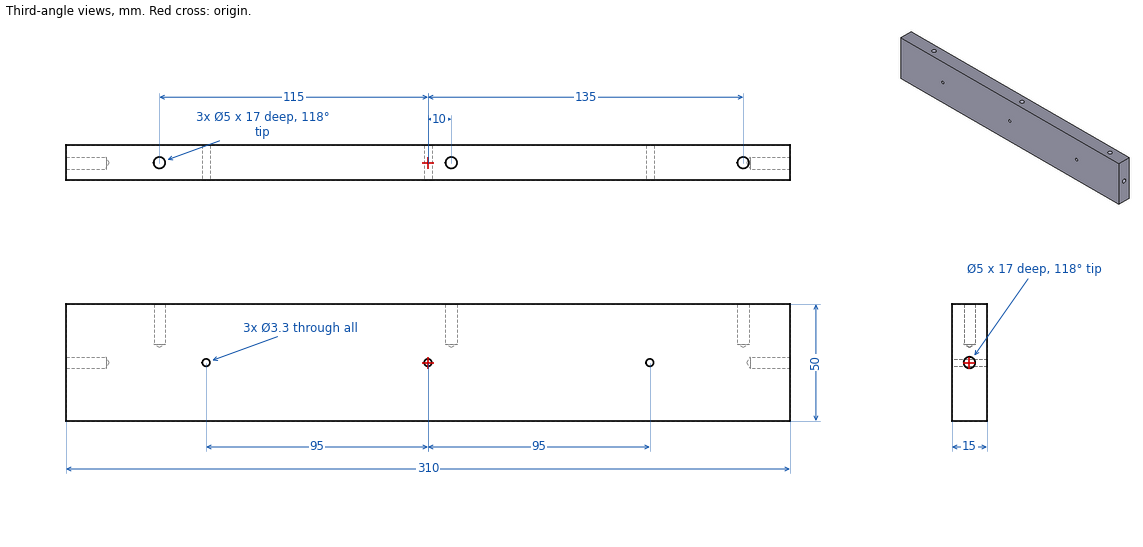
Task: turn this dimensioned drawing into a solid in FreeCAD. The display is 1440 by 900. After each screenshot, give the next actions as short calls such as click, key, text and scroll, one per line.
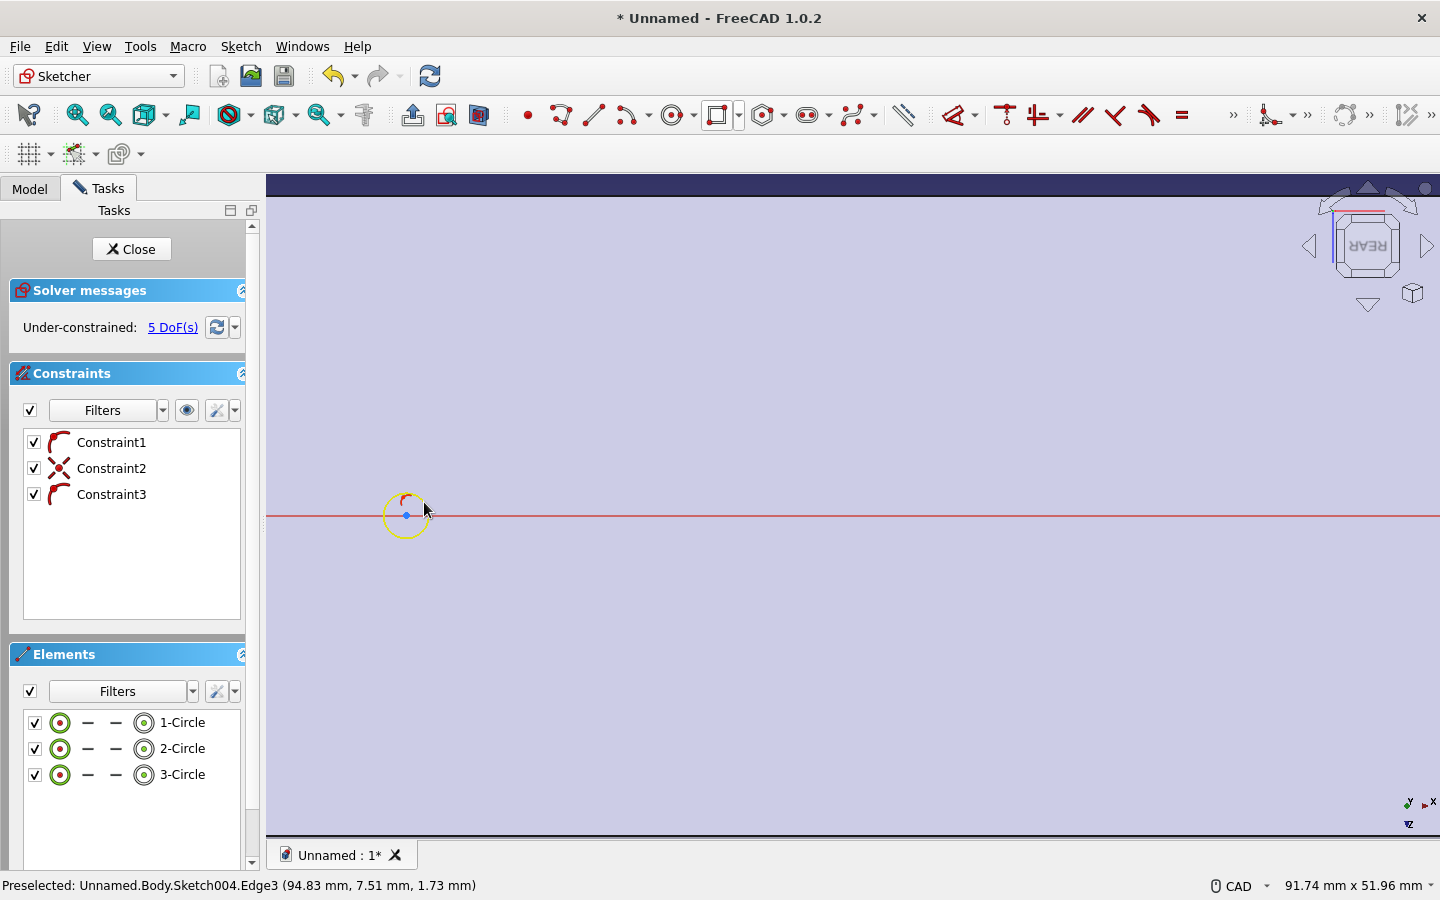
click(422, 500)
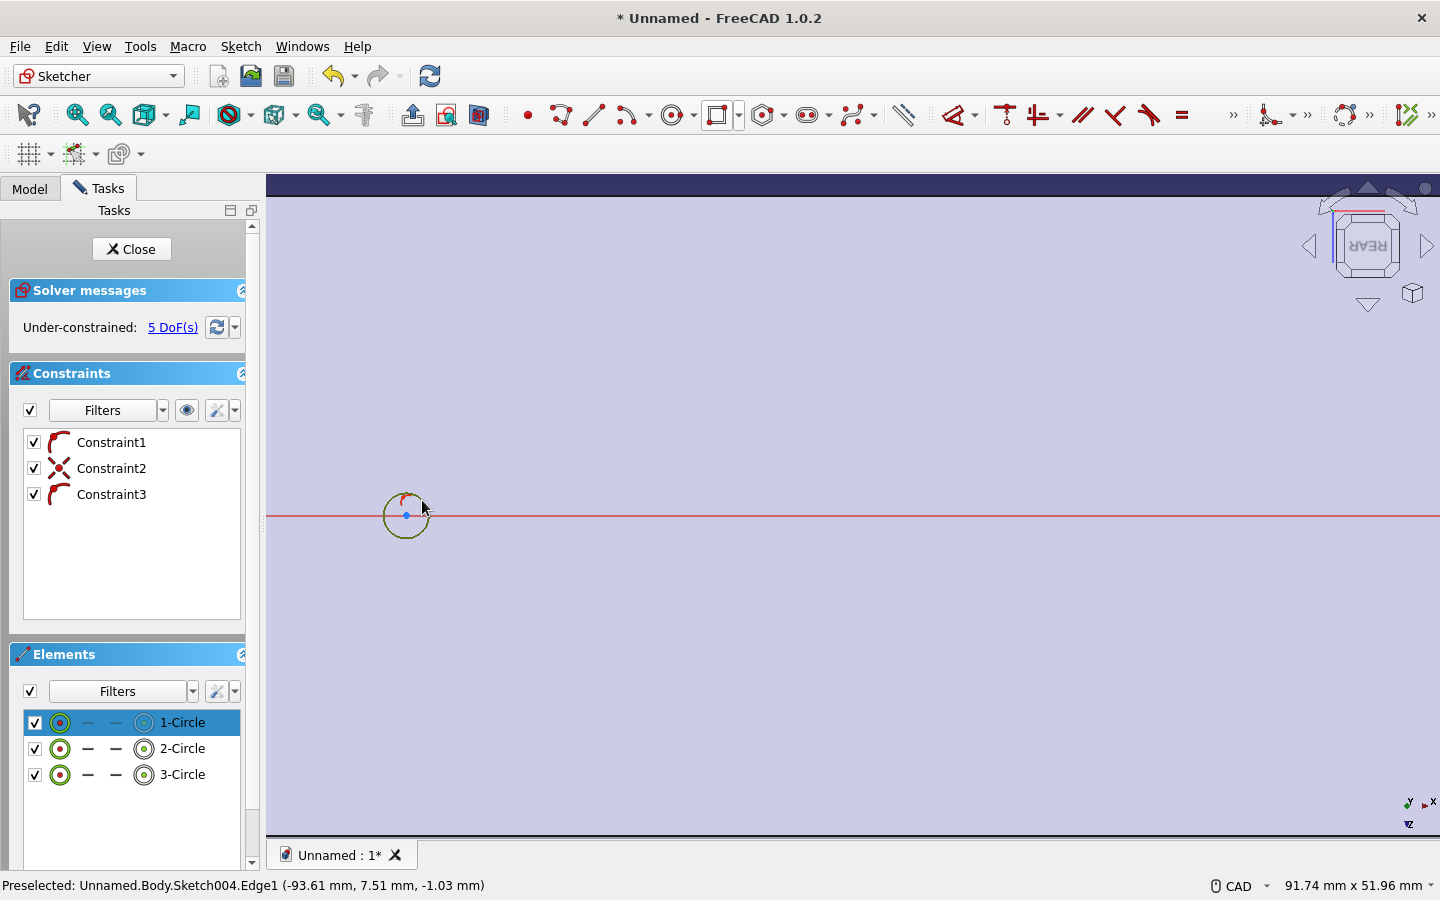
scroll(423, 502, down, 6)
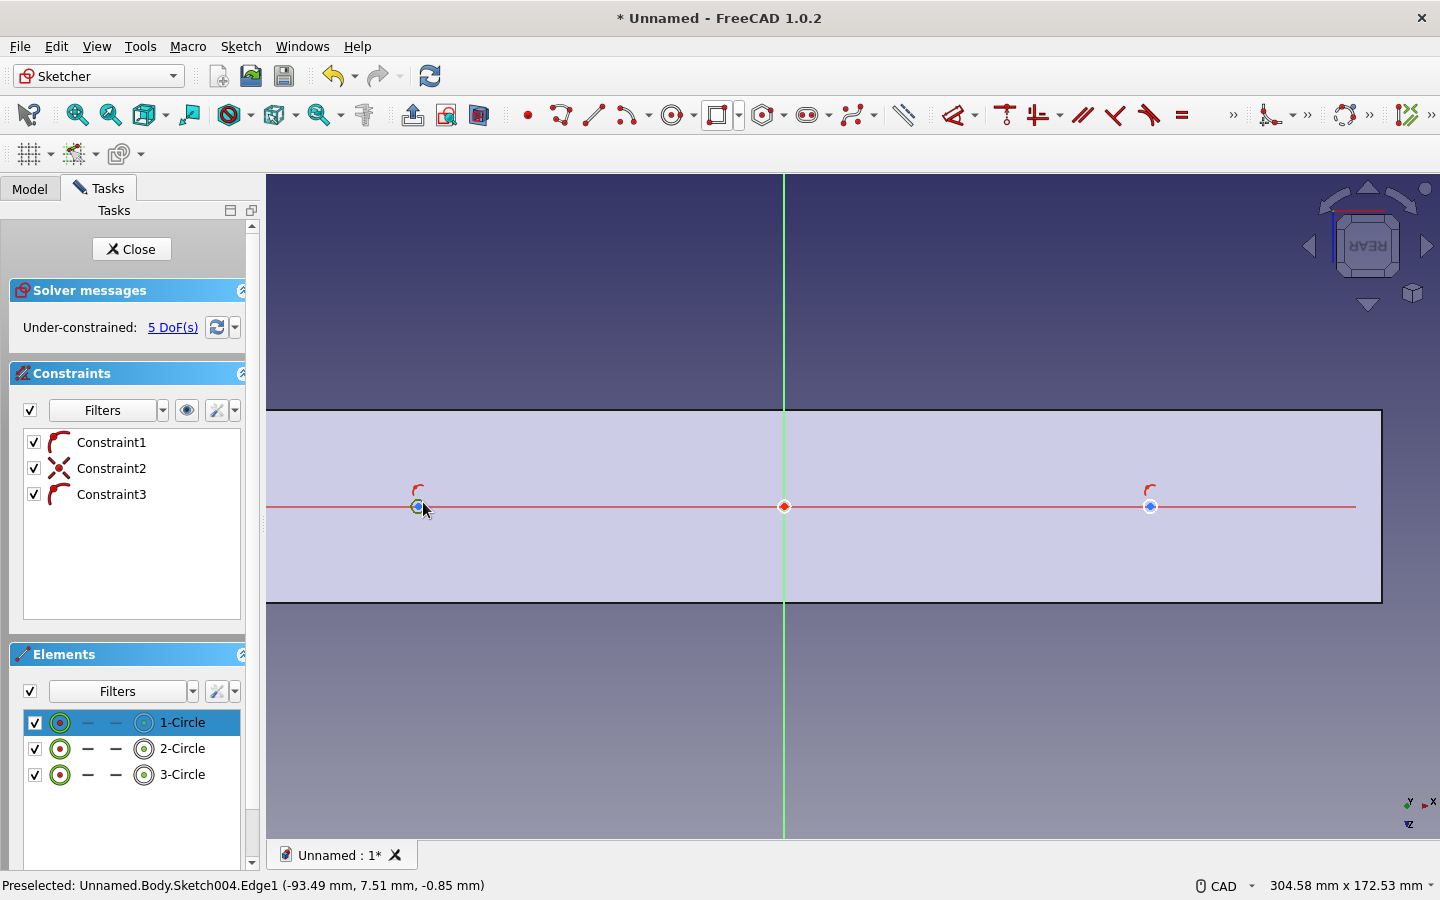
scroll(789, 502, up, 6)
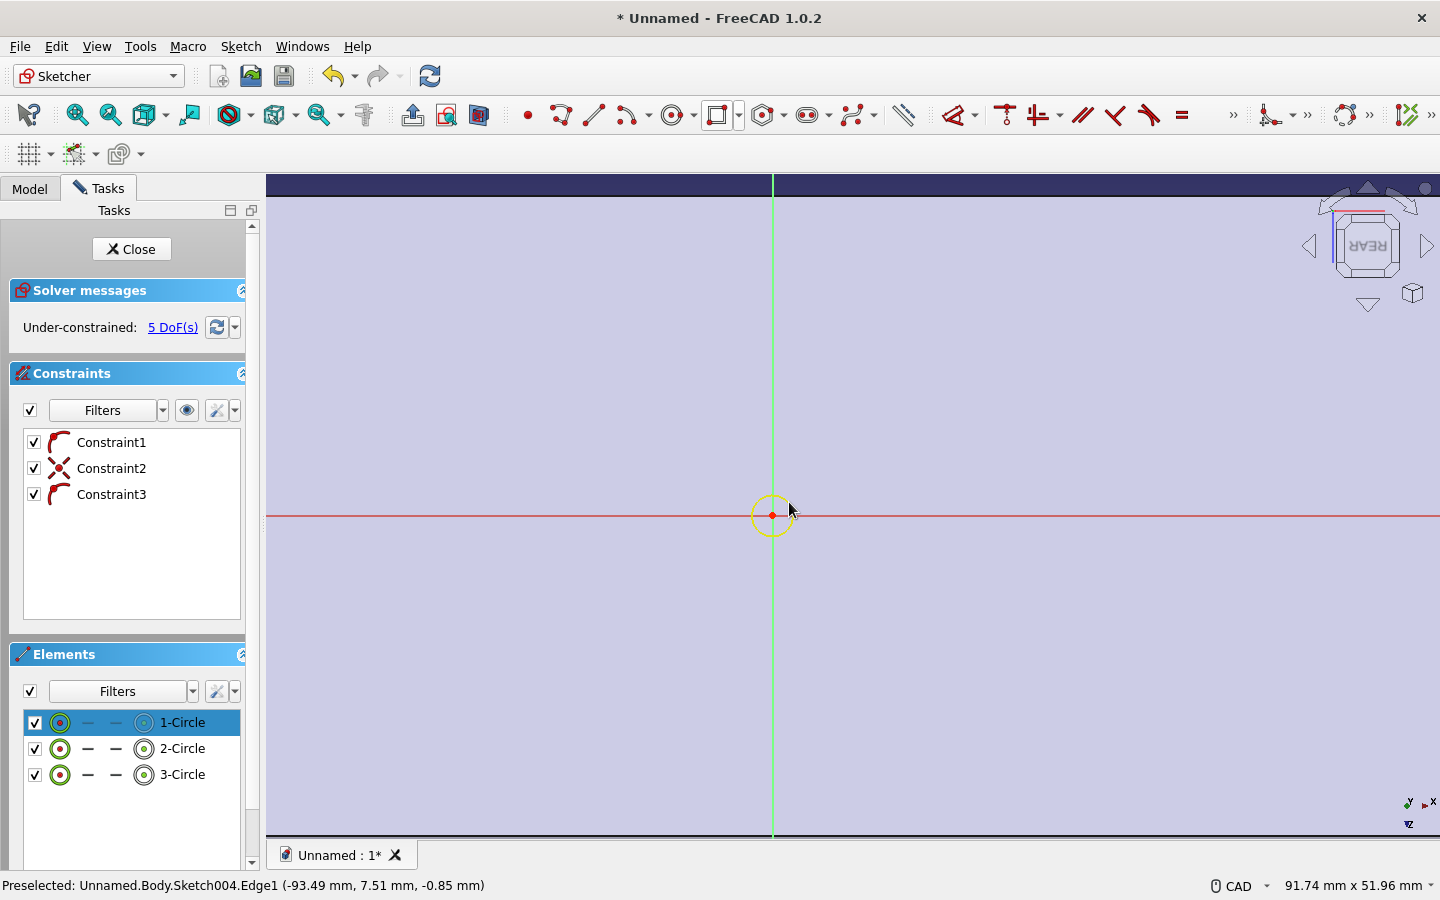
click(787, 501)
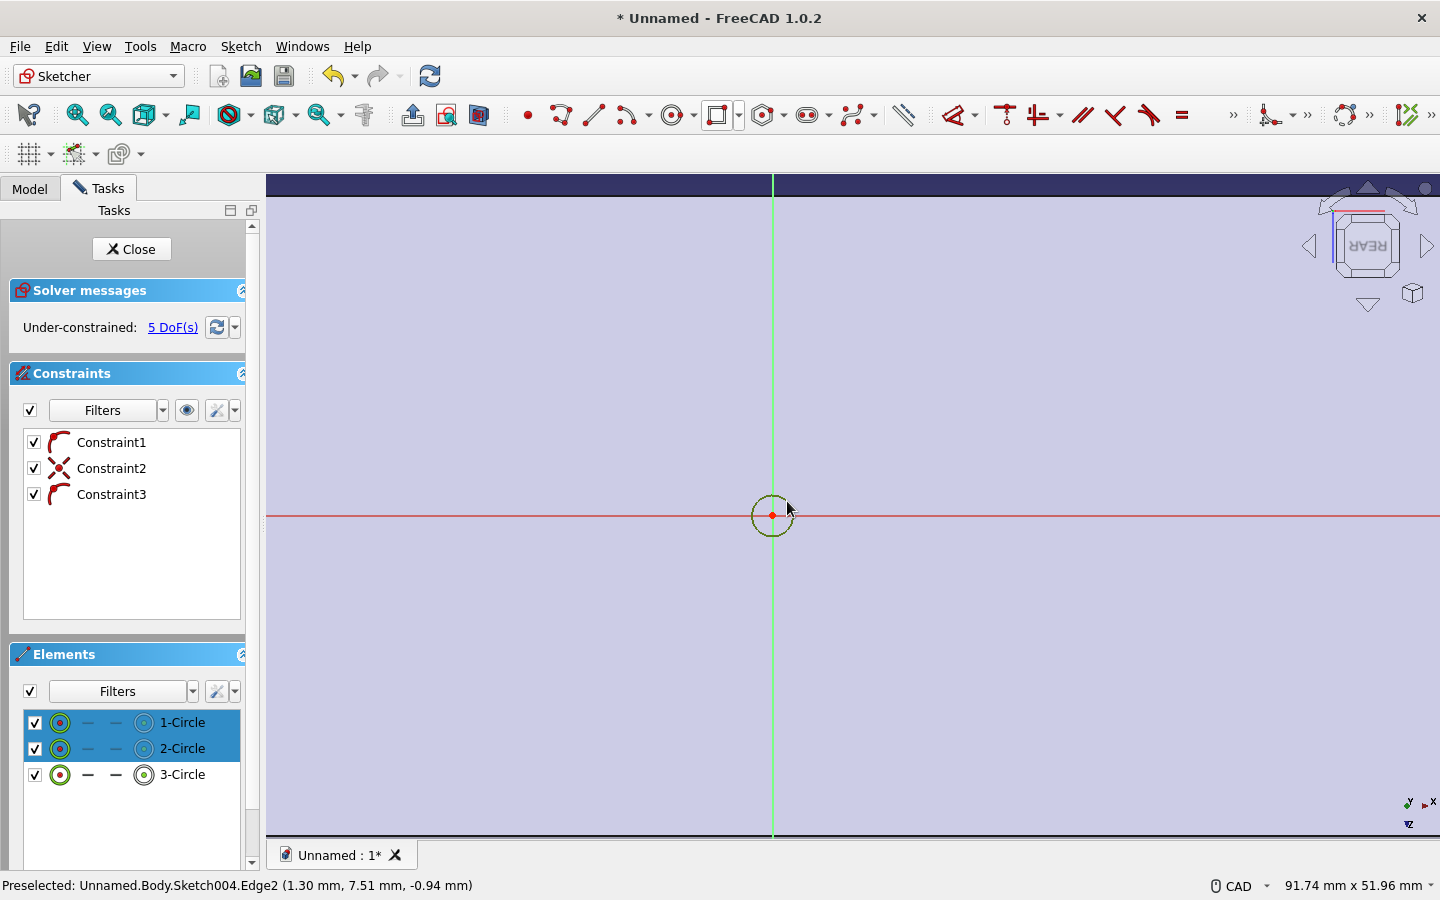
scroll(790, 502, down, 6)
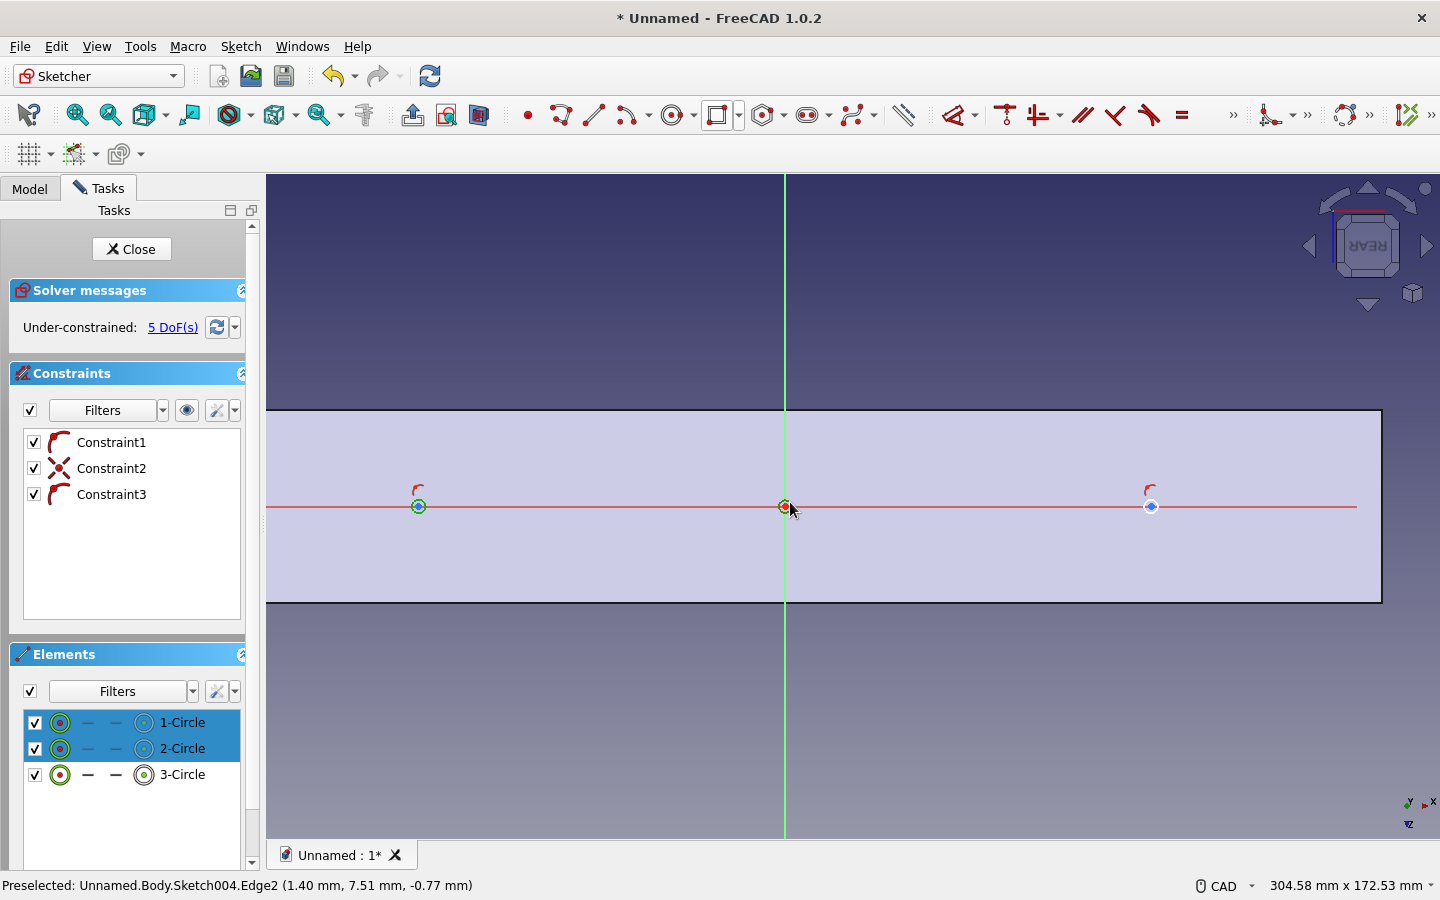
scroll(1156, 502, up, 6)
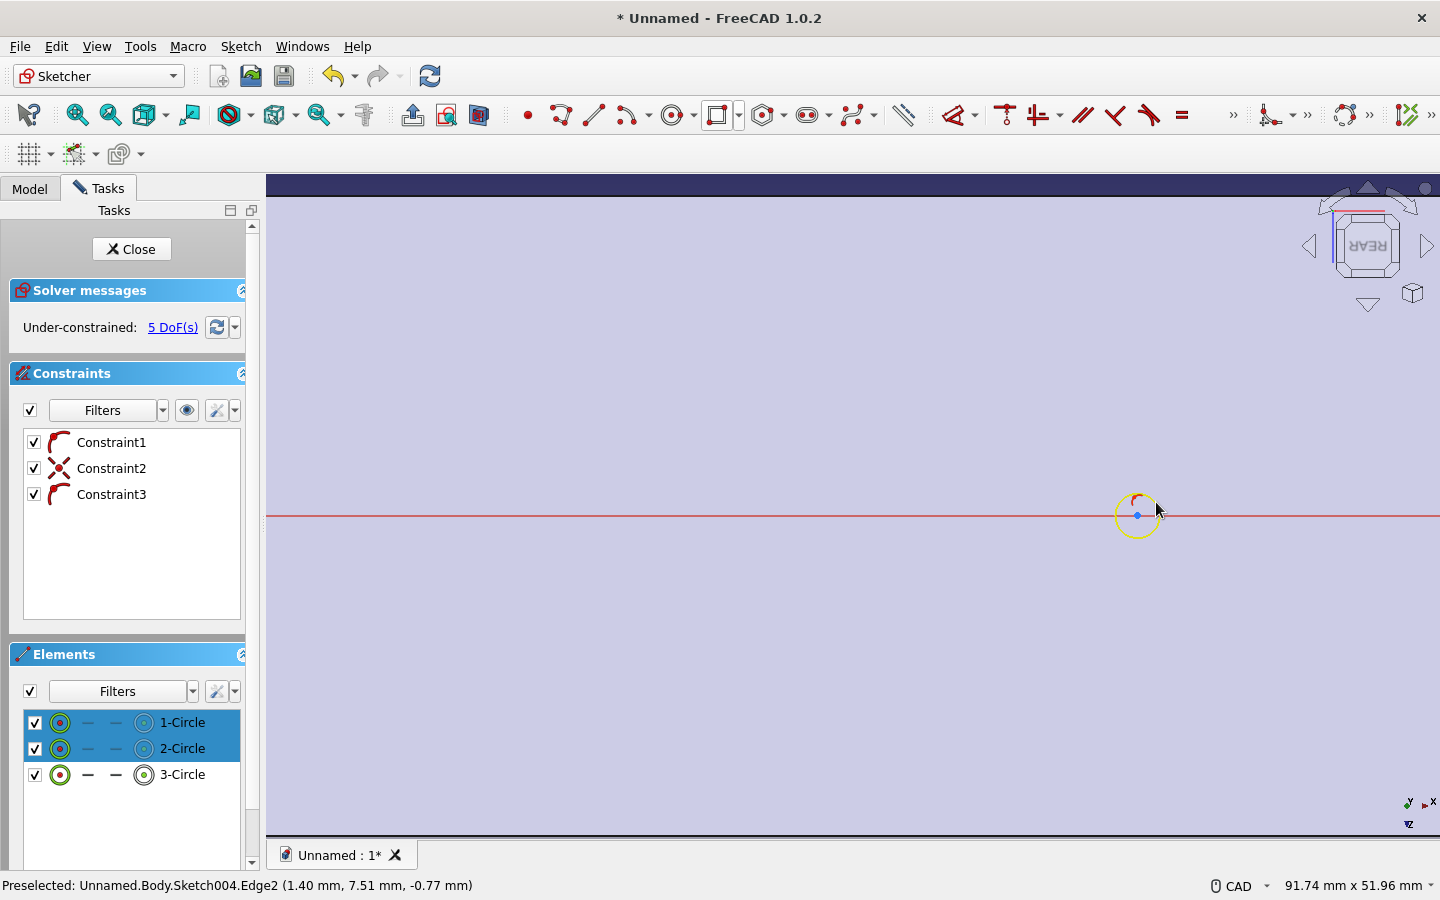
click(1153, 500)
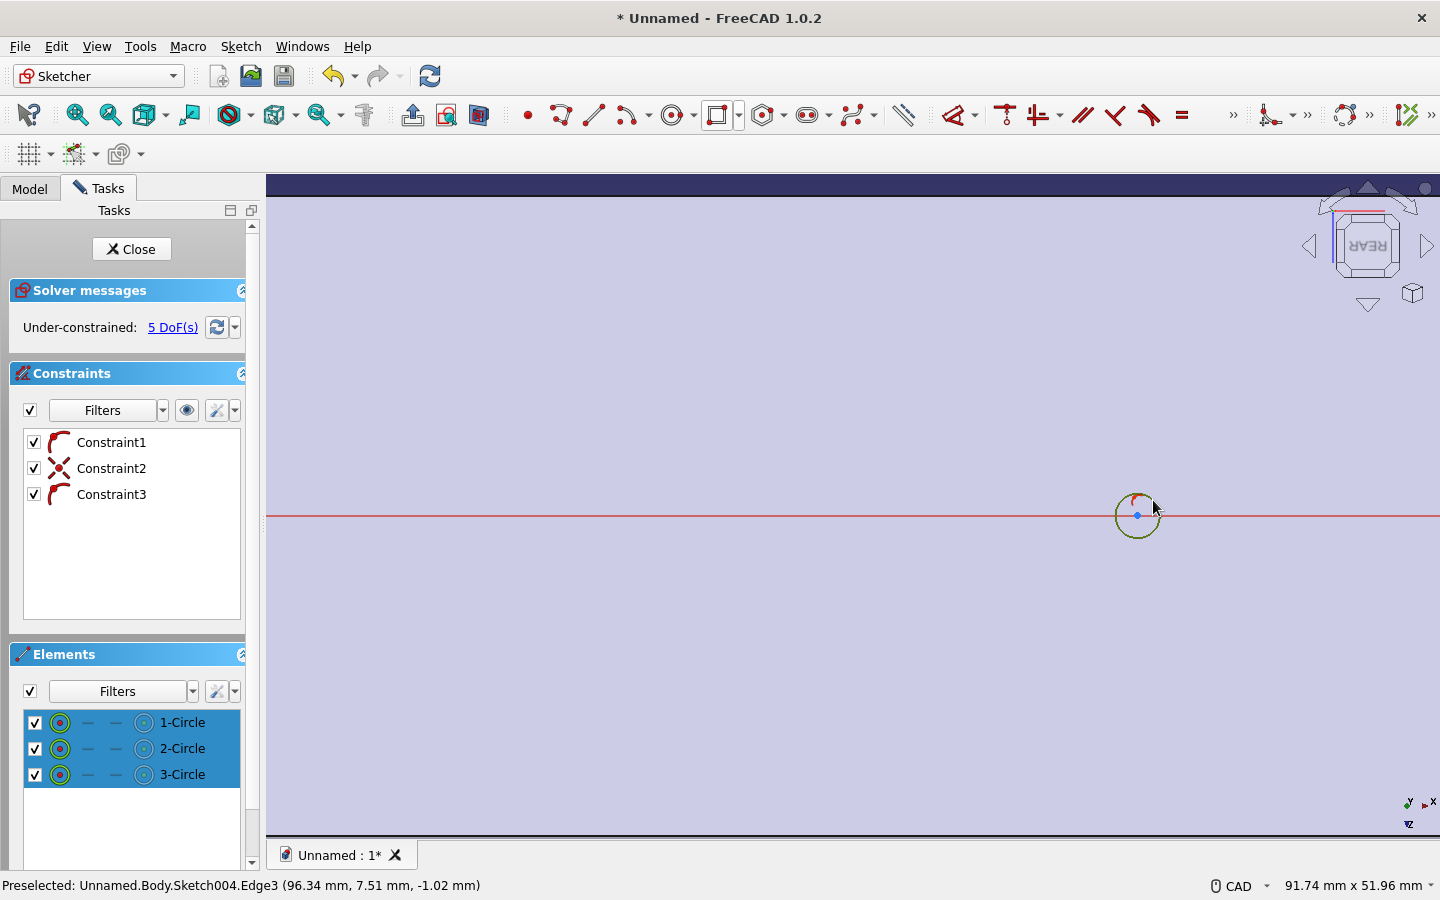
click(1182, 116)